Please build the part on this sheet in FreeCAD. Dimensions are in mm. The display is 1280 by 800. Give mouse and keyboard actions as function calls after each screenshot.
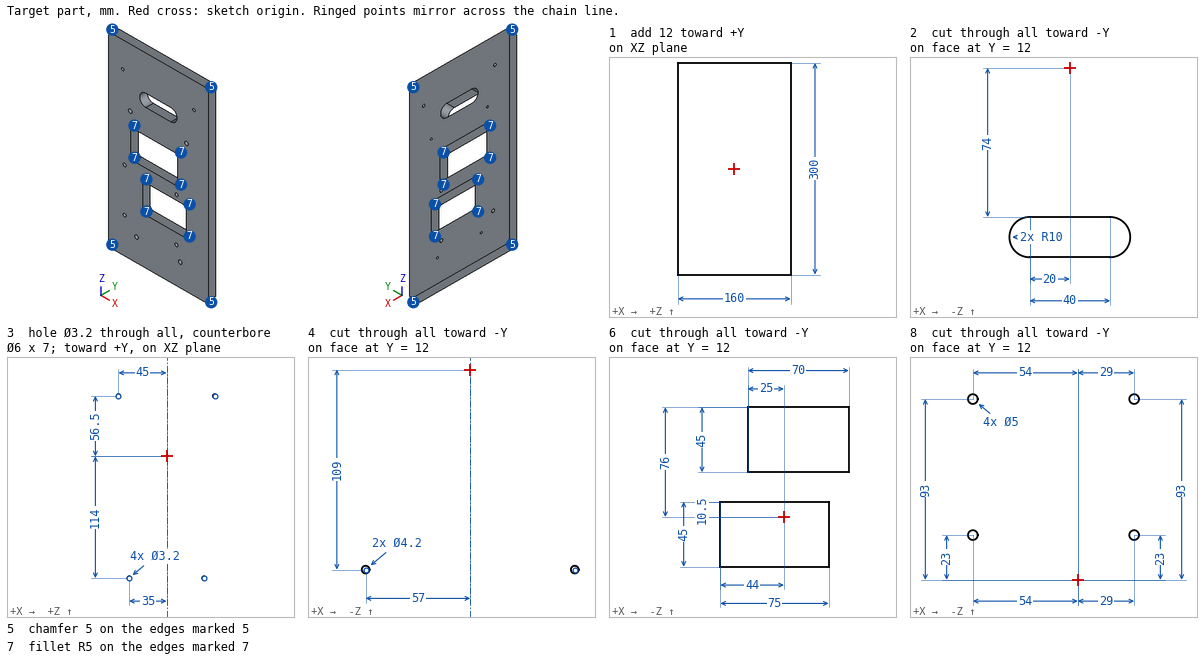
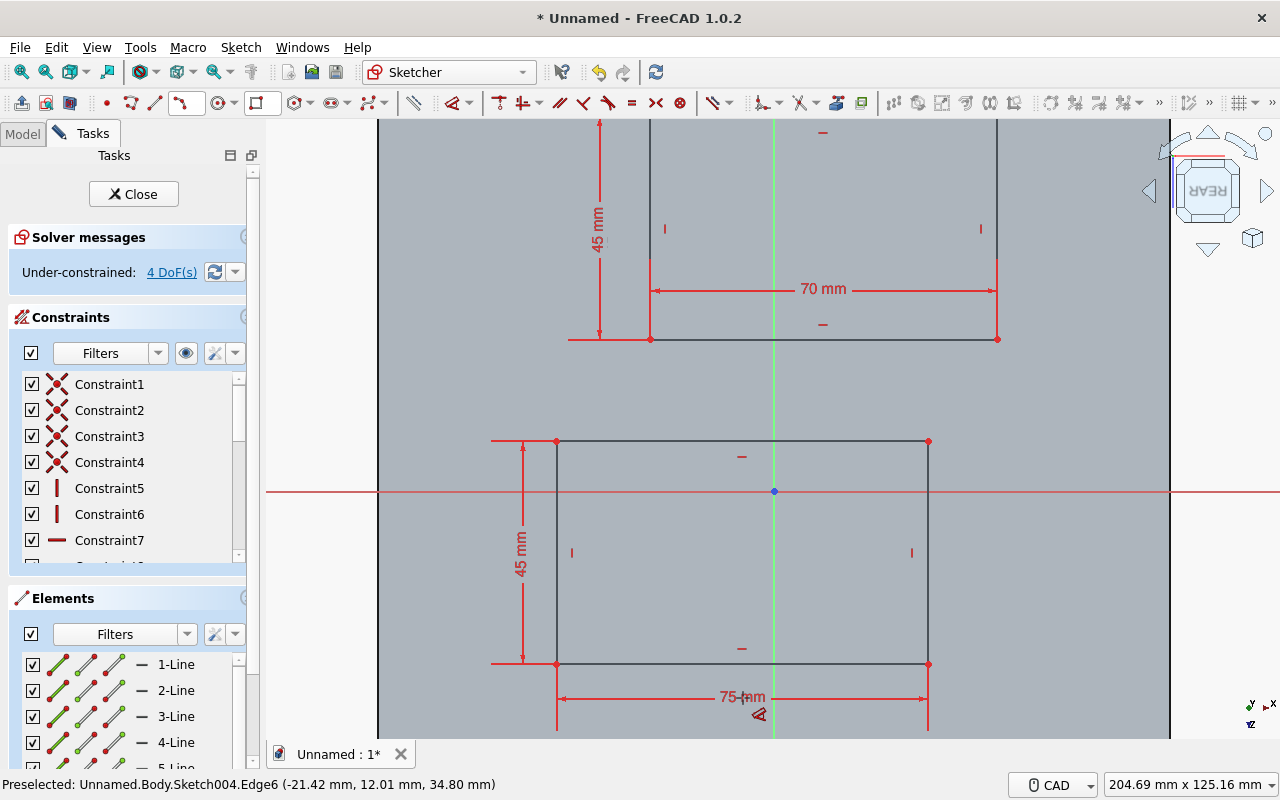
scroll(558, 510, down, 2)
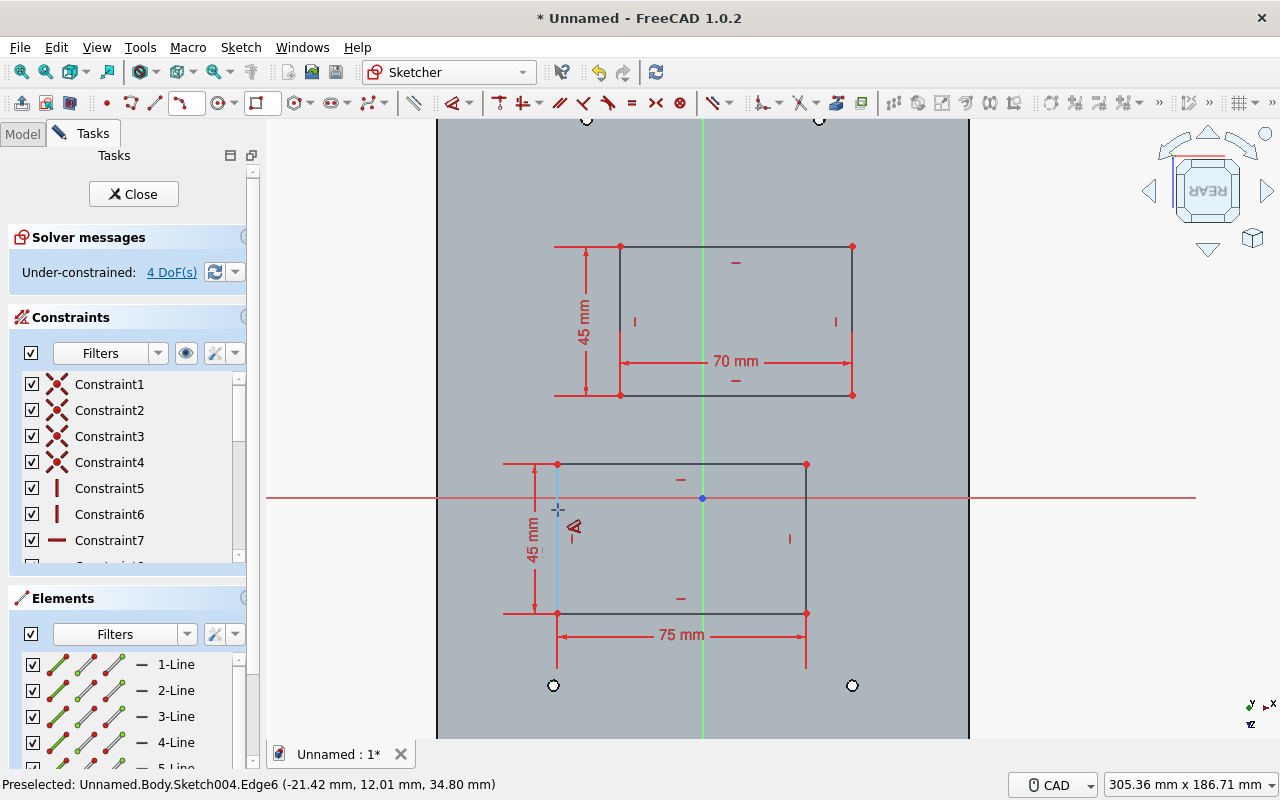
click(620, 247)
click(662, 213)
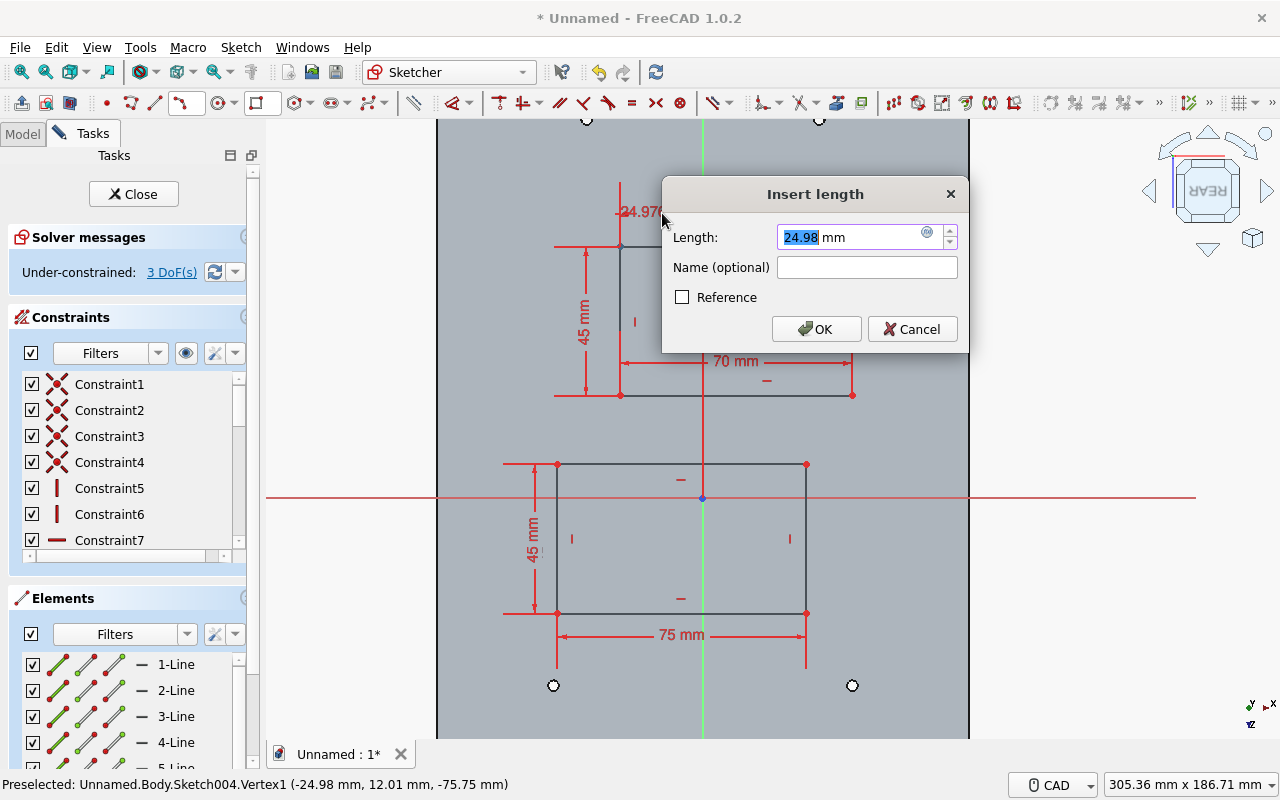
text(25)
key(Return)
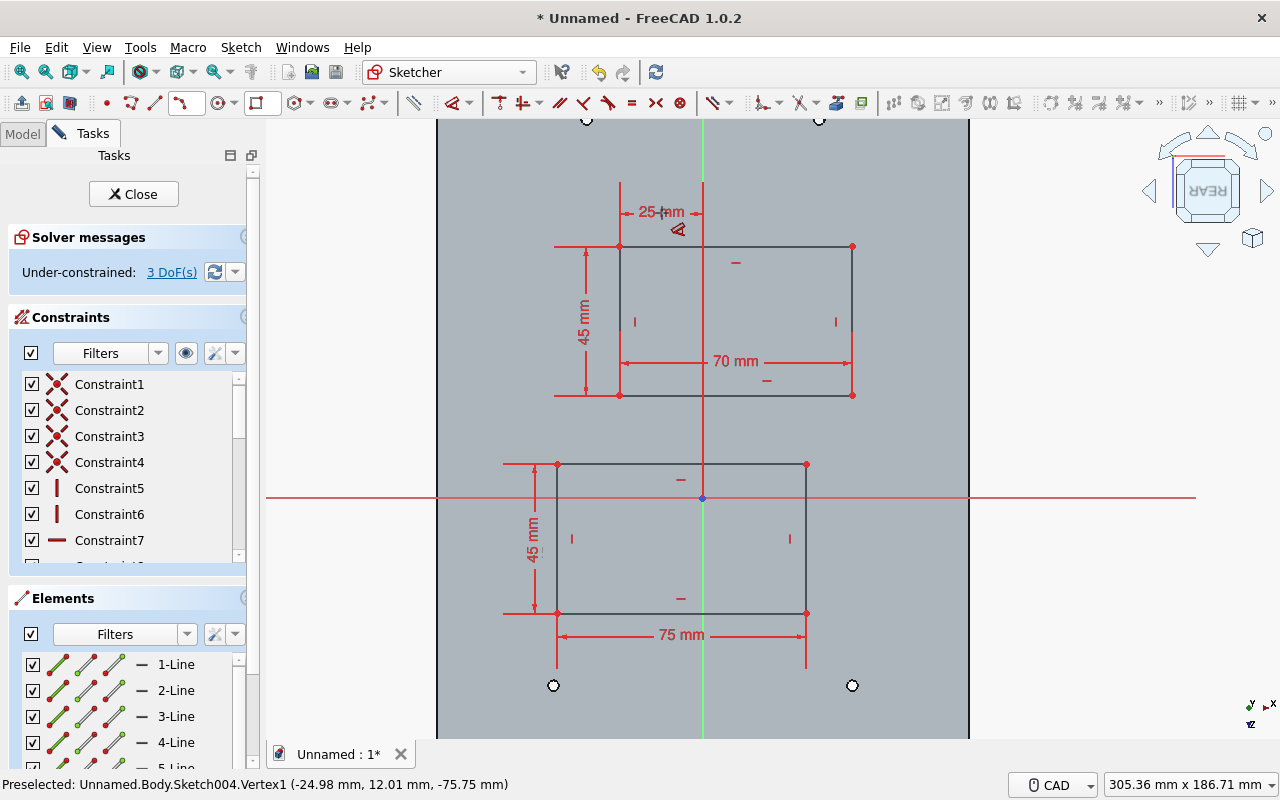
click(620, 247)
click(586, 372)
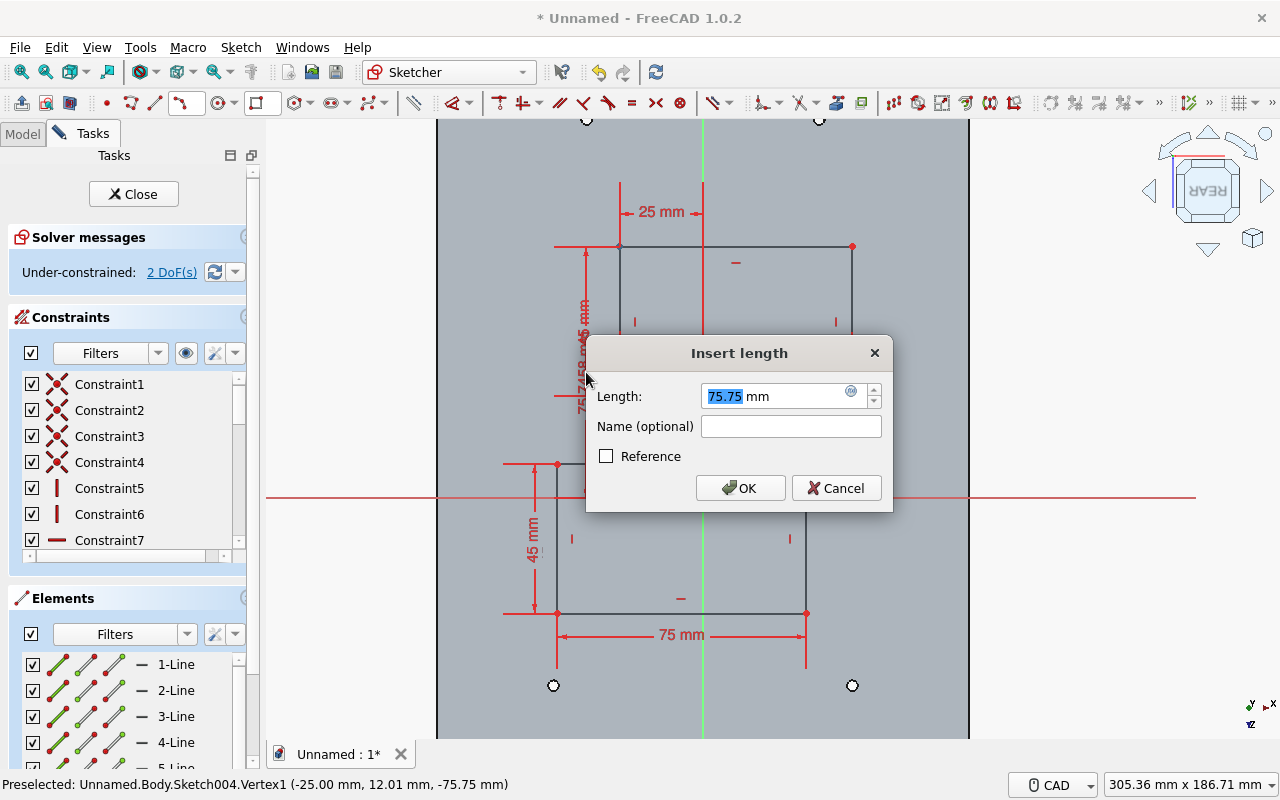
text(76)
key(Return)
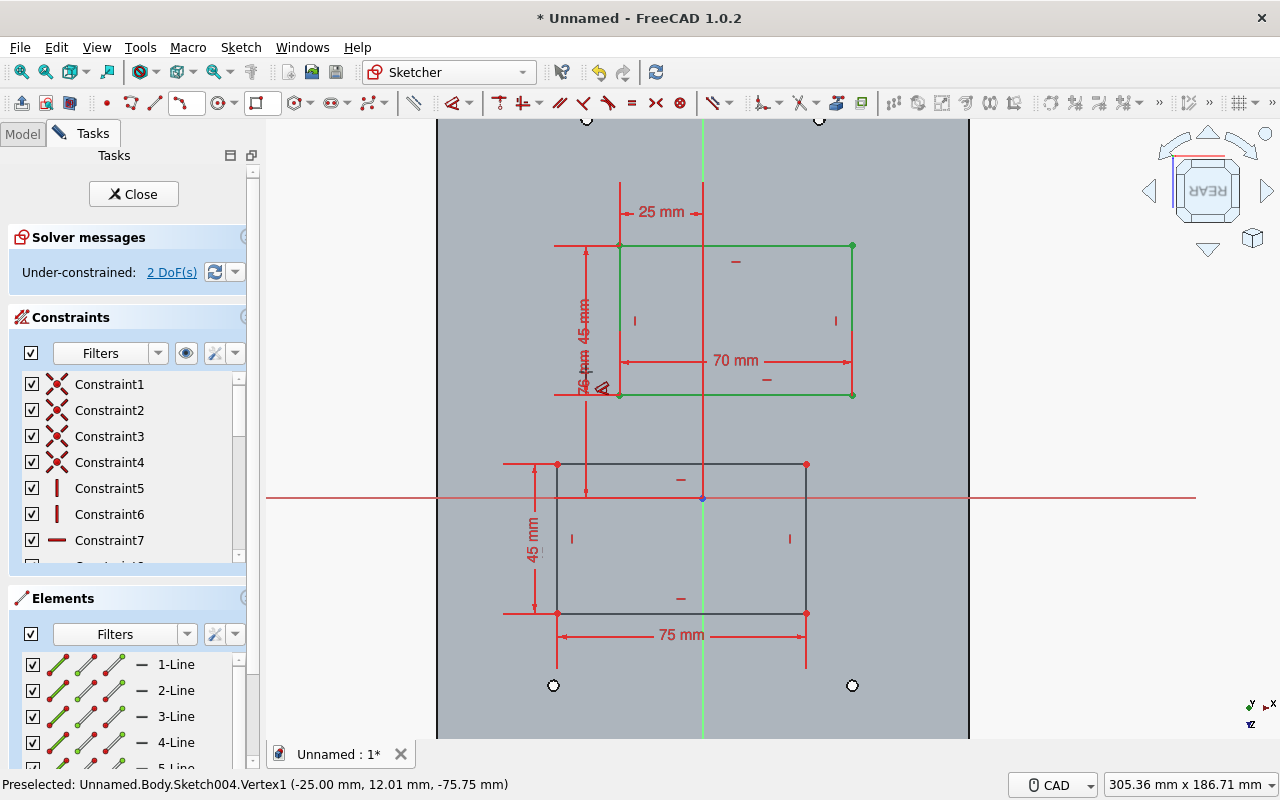
click(557, 464)
click(630, 532)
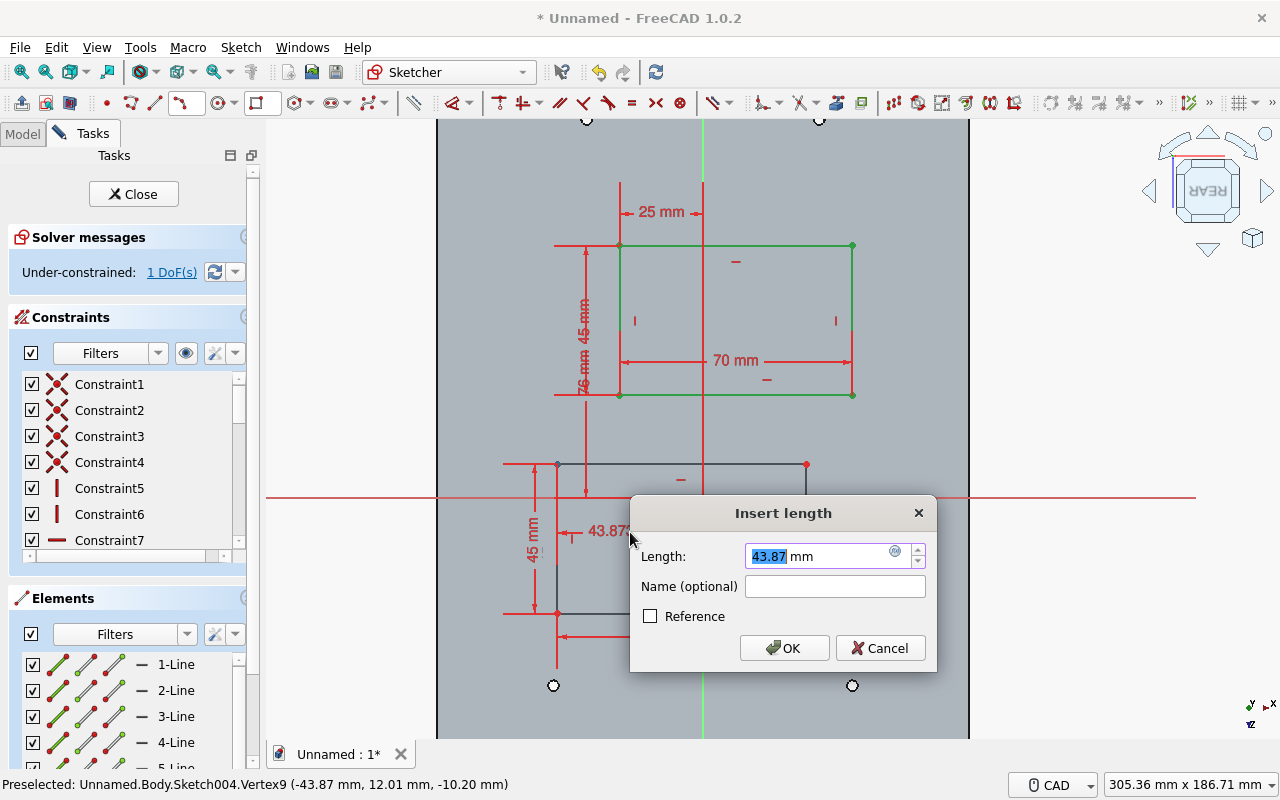
text(44)
key(Return)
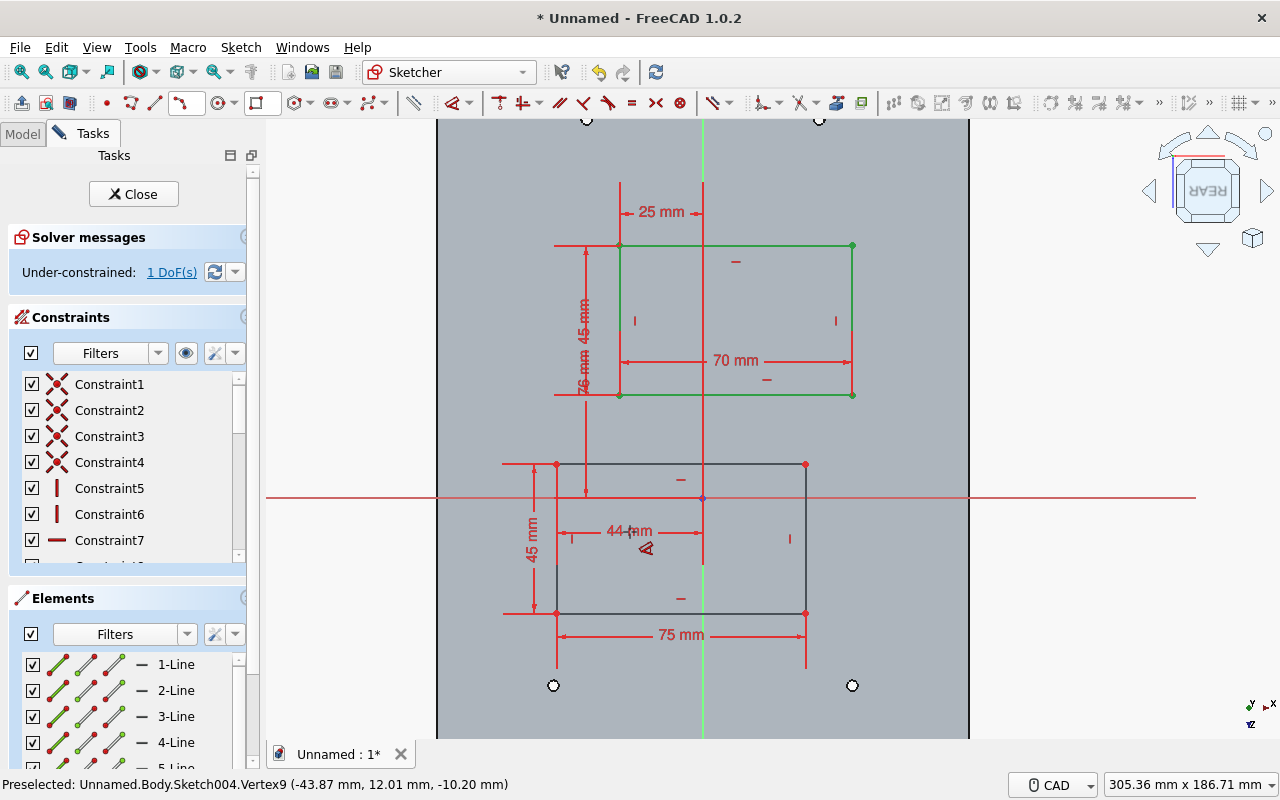
click(557, 464)
click(523, 481)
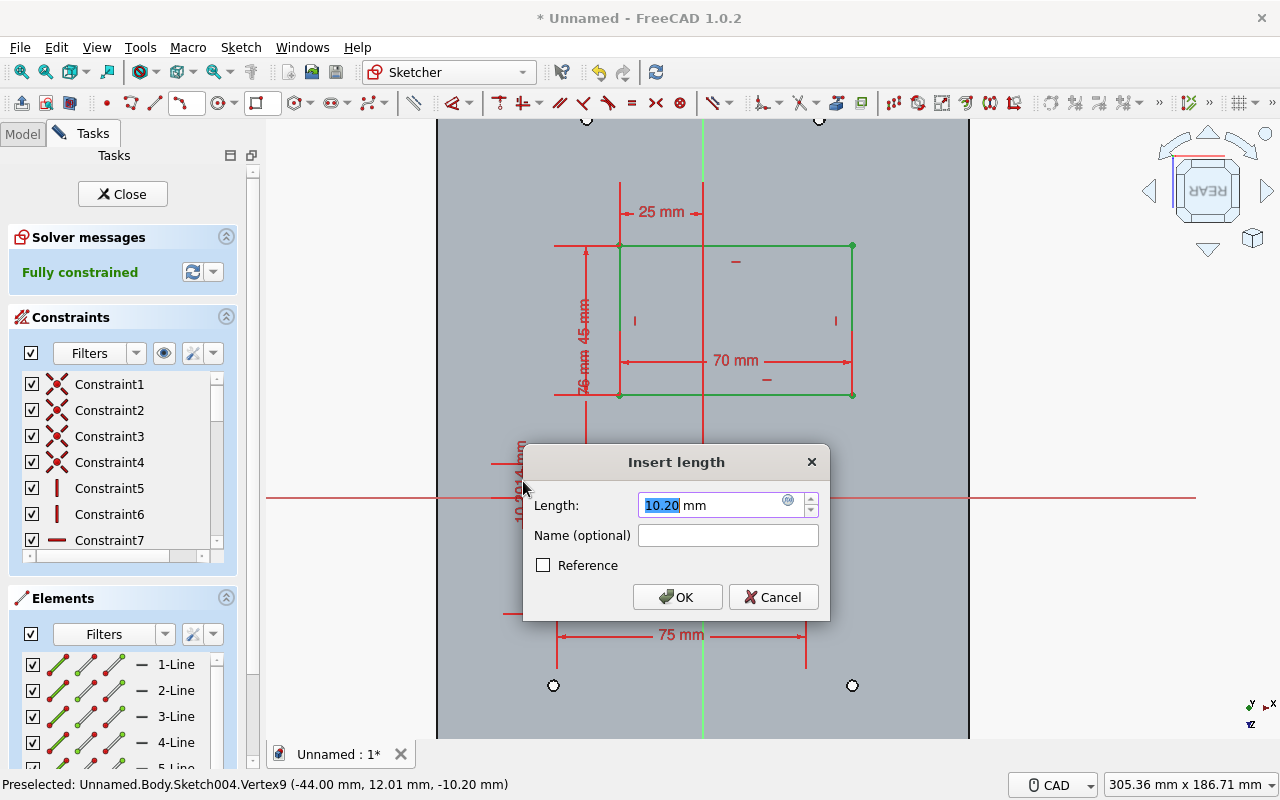
text(10.5)
key(Return)
key(Escape)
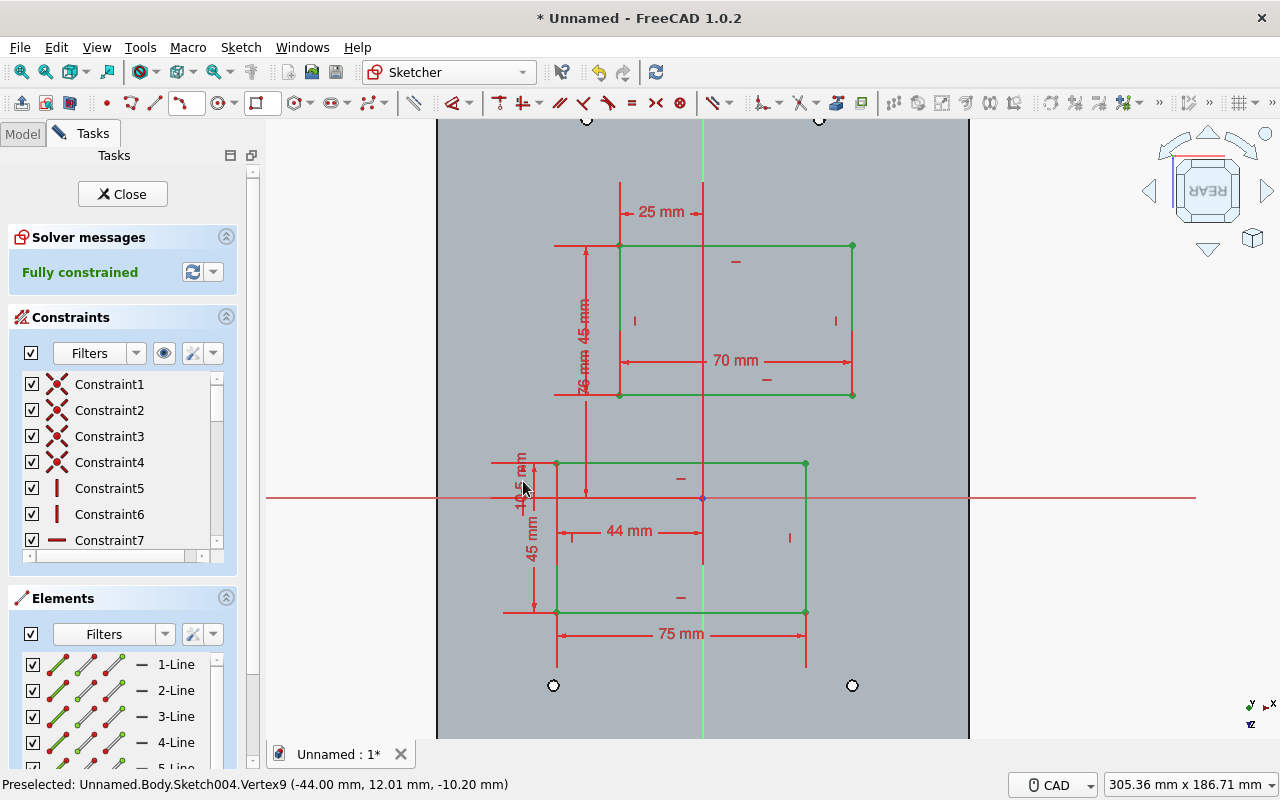
click(123, 194)